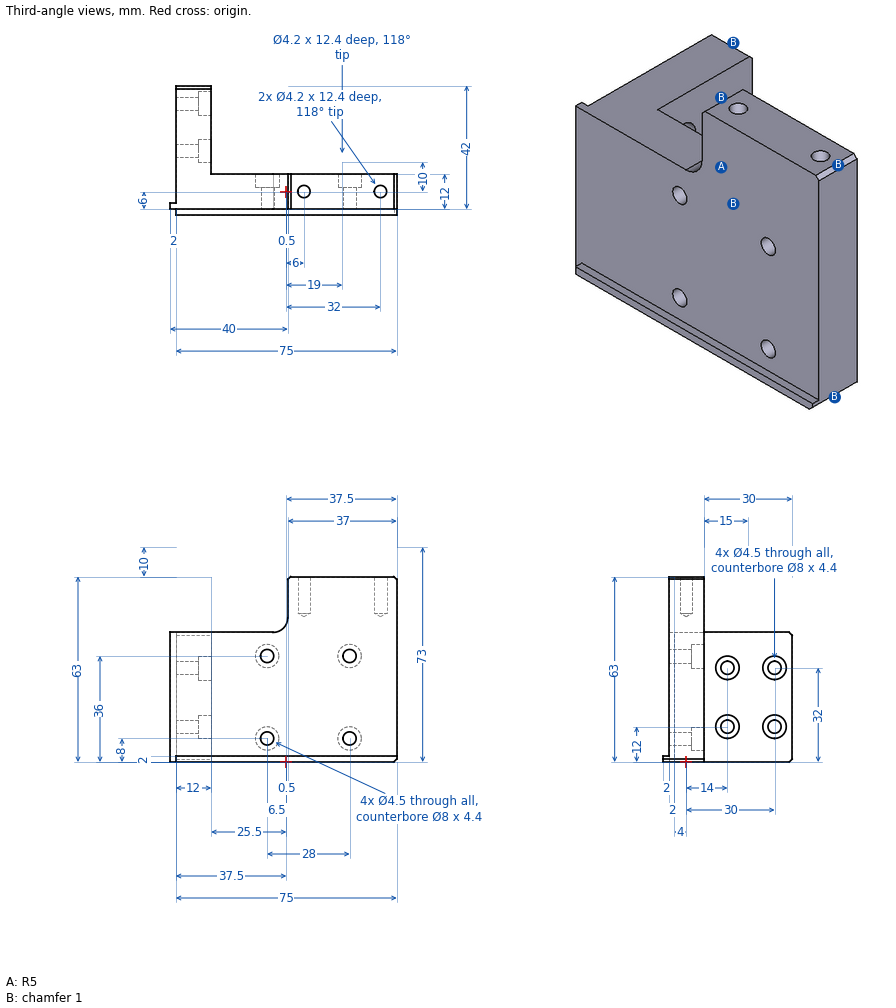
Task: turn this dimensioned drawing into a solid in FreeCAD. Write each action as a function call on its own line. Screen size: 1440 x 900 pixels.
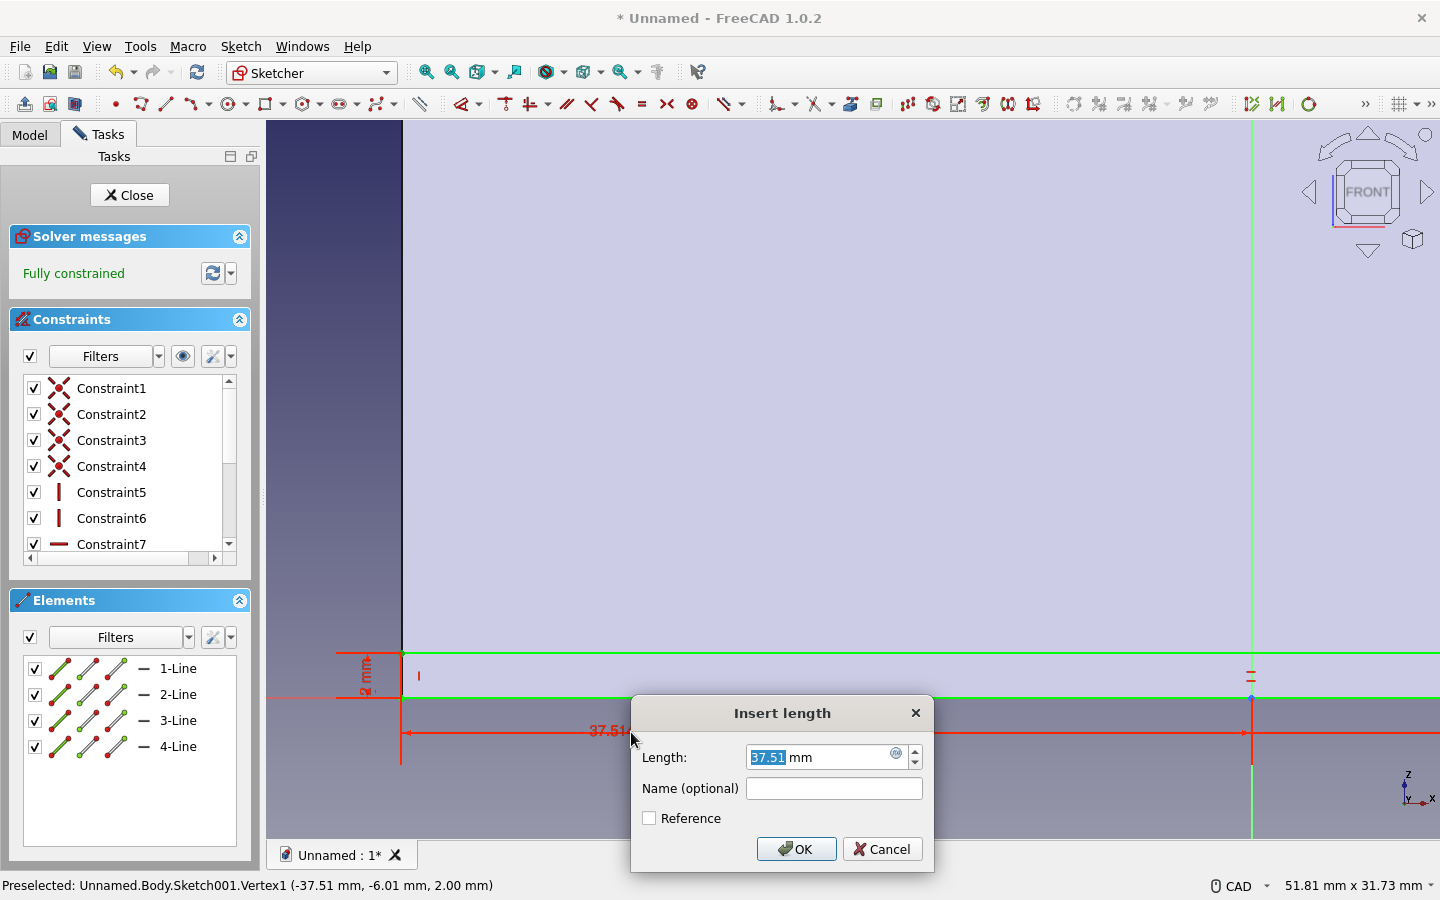
text(37.5)
key(Return)
key(Escape)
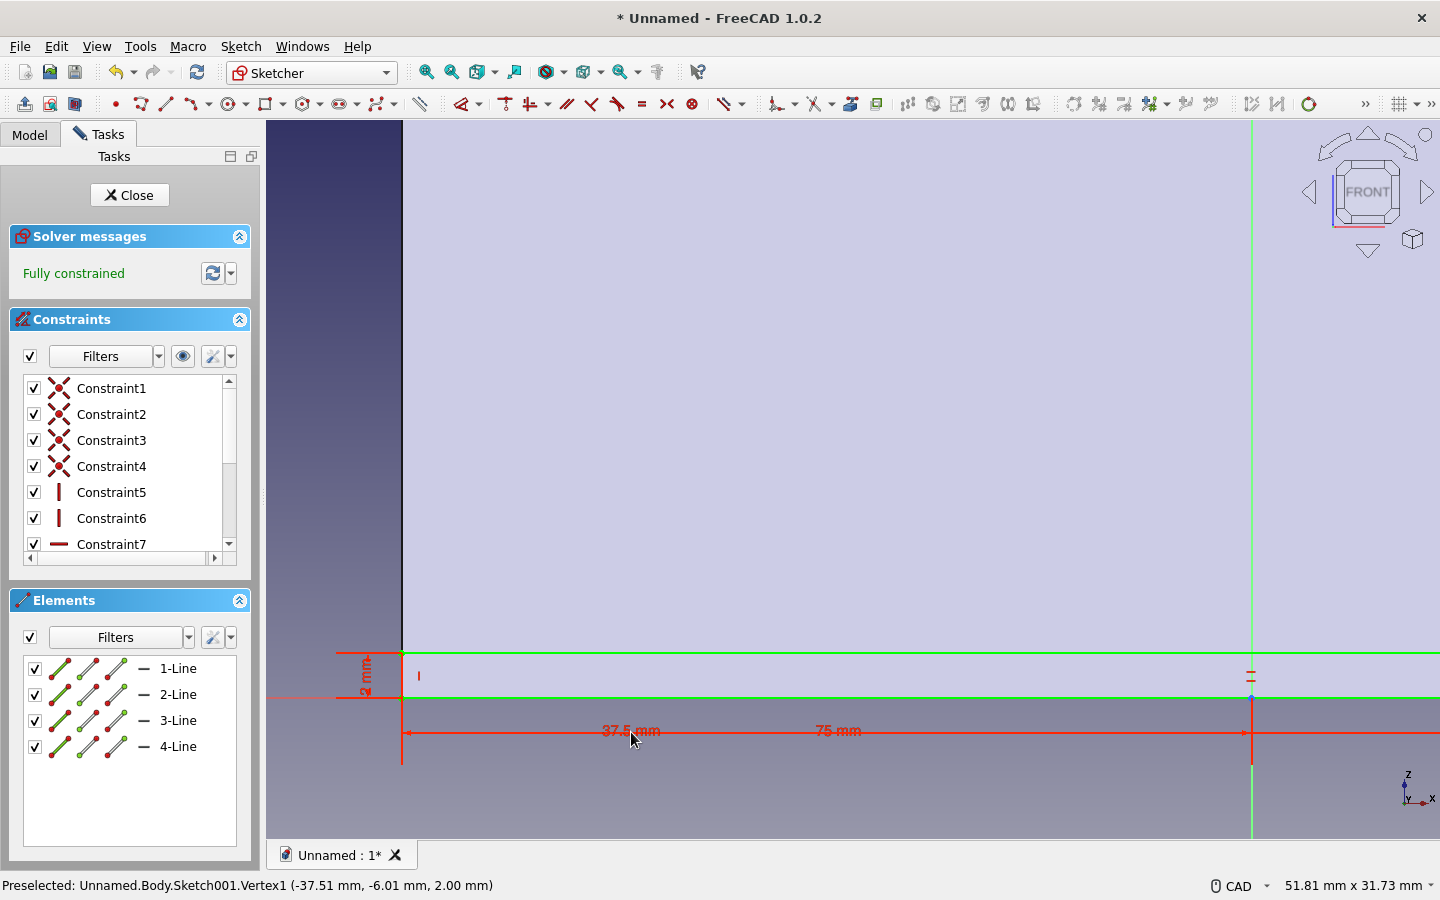
click(130, 195)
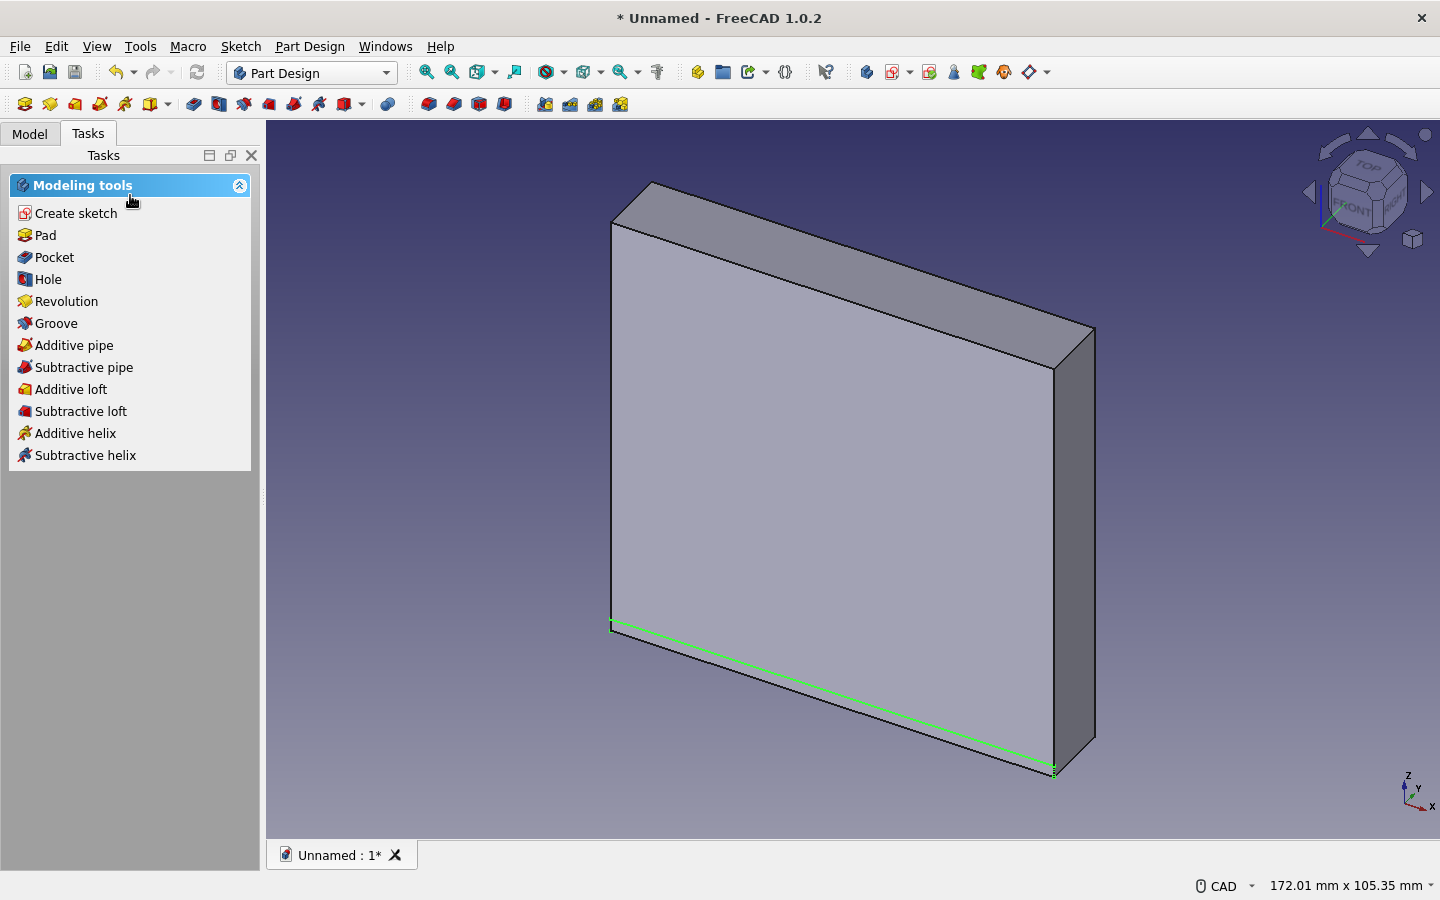
click(25, 104)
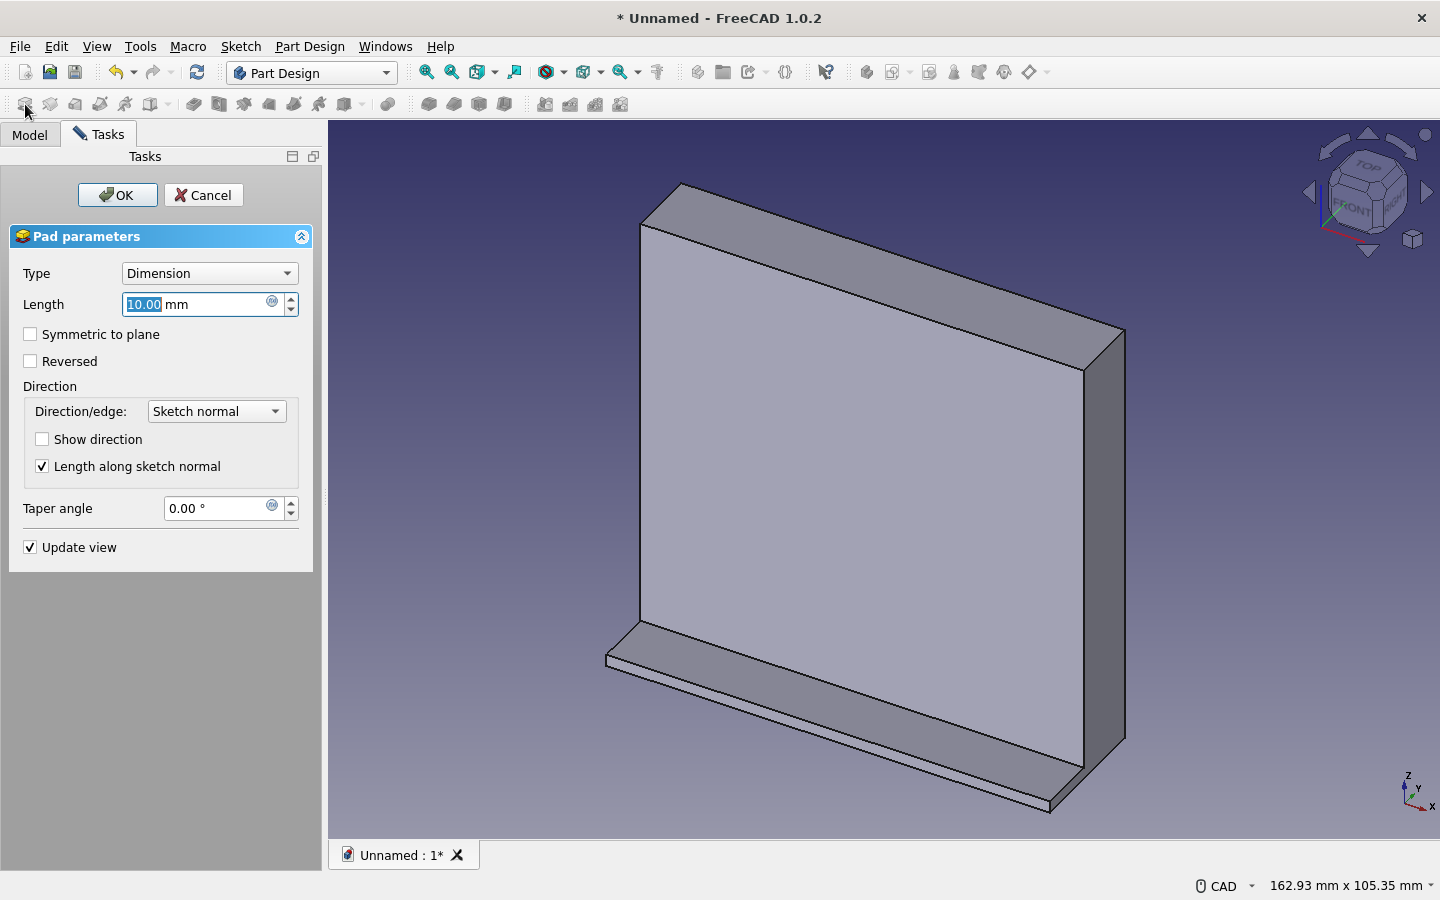
text(2)
key(Tab)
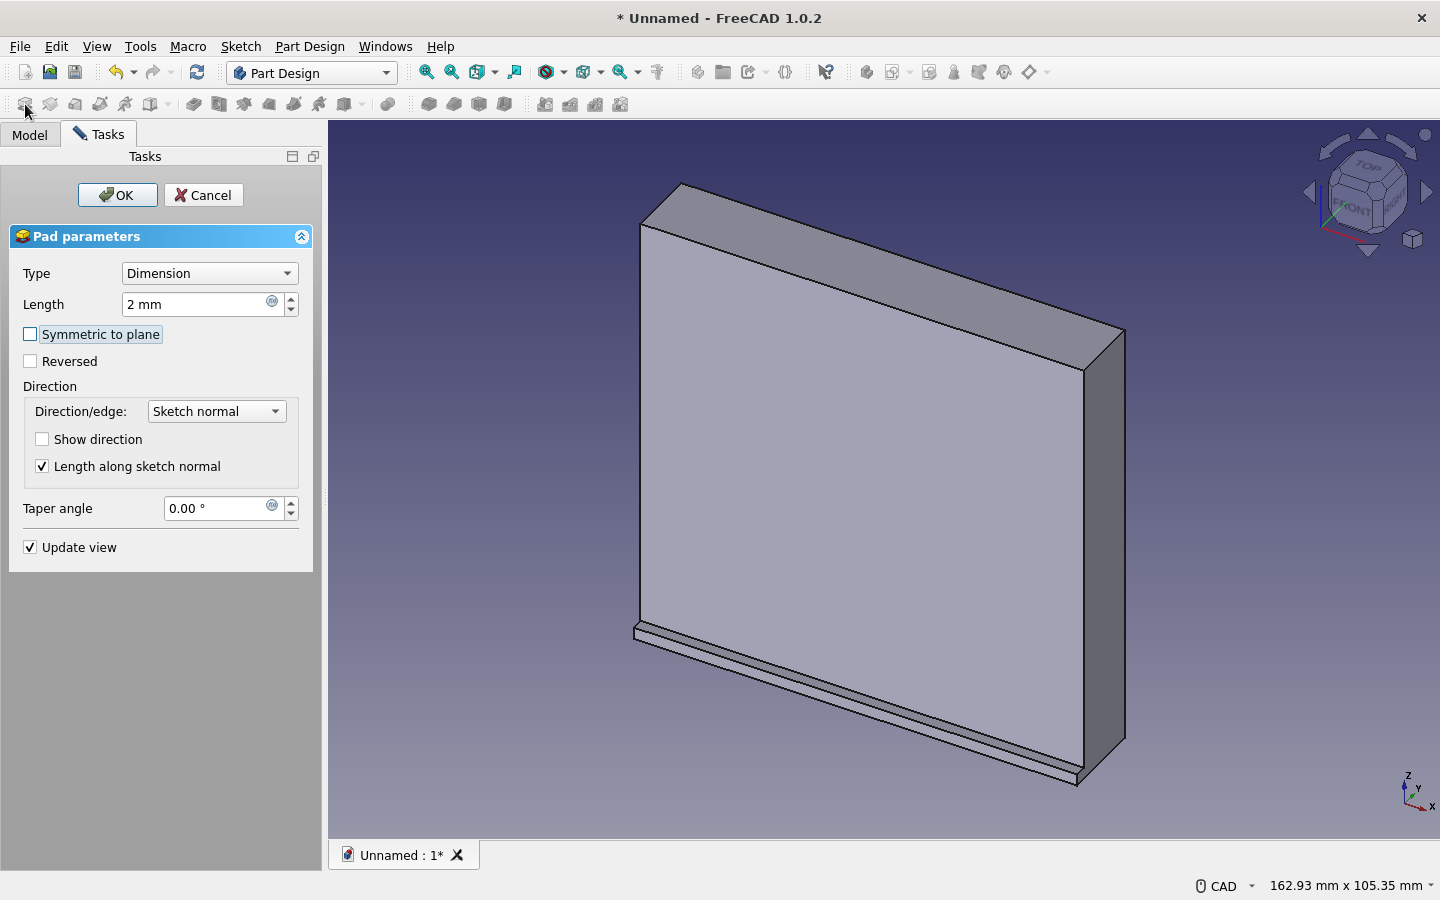
click(118, 195)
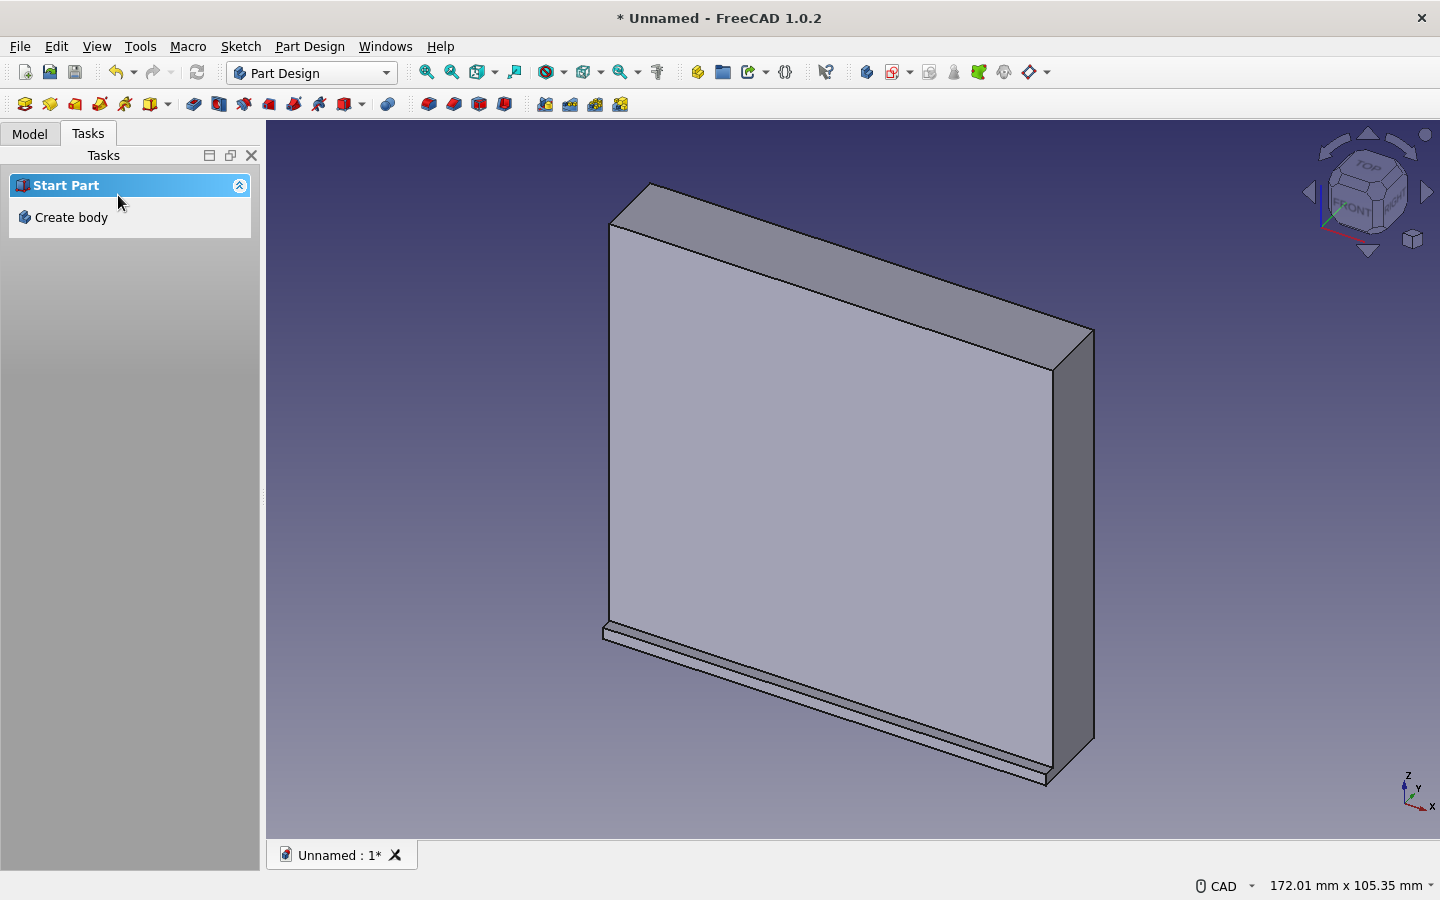
key(4)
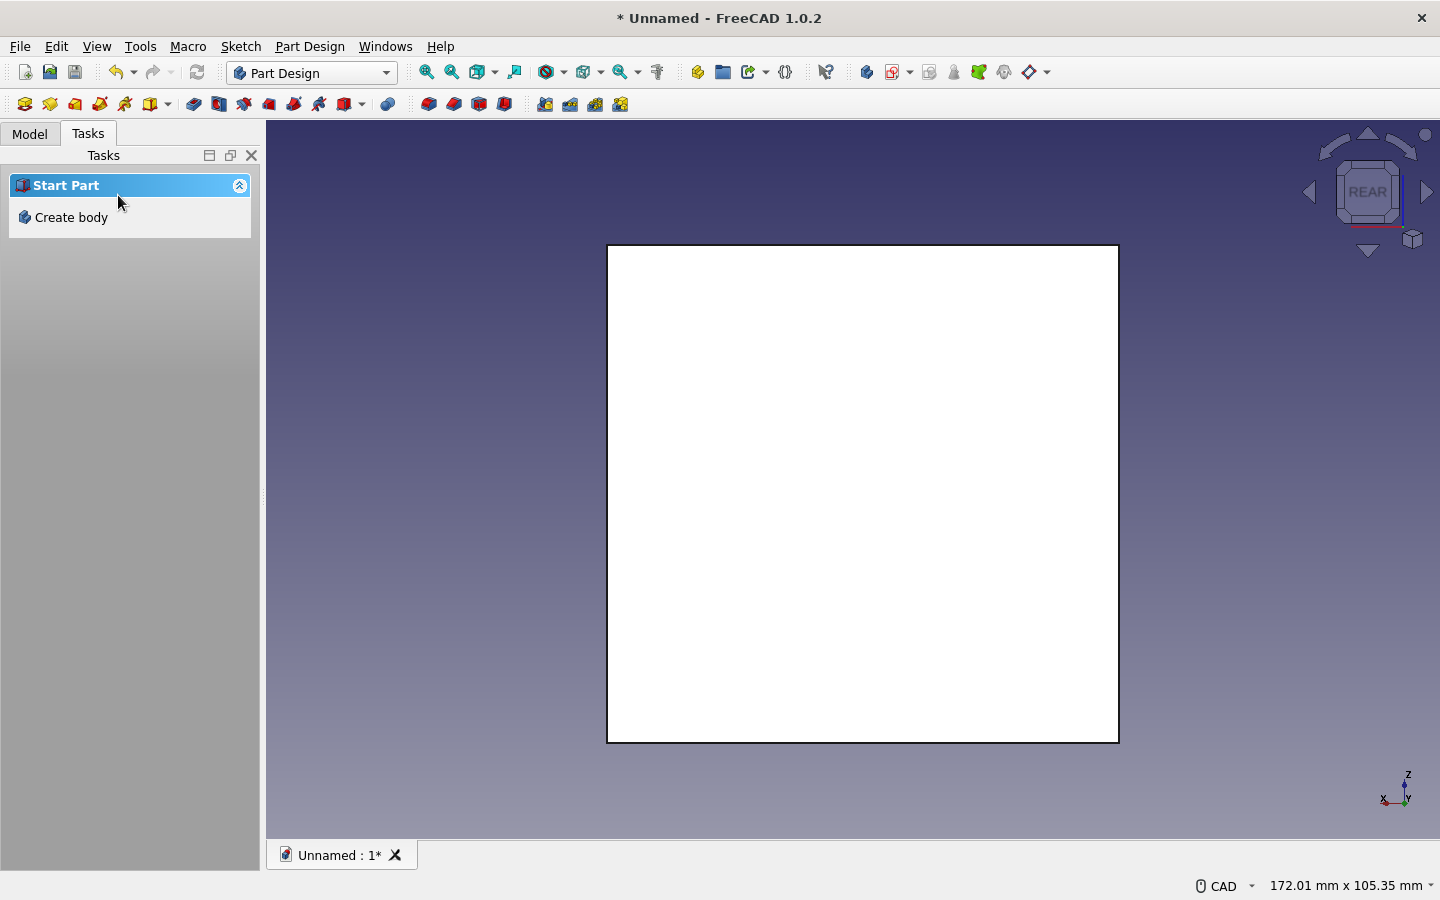
click(863, 493)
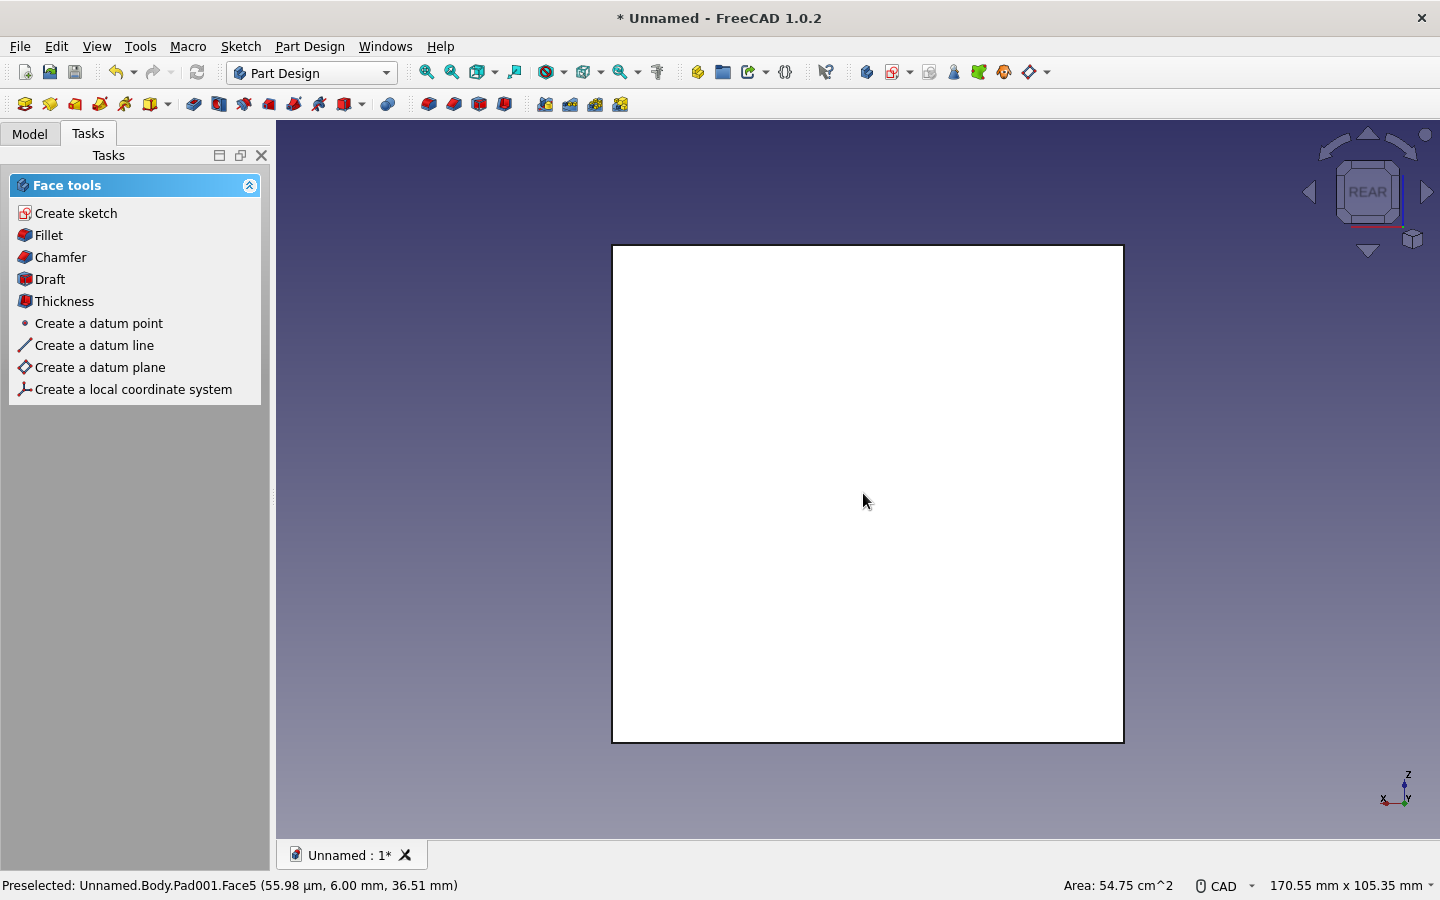
click(892, 72)